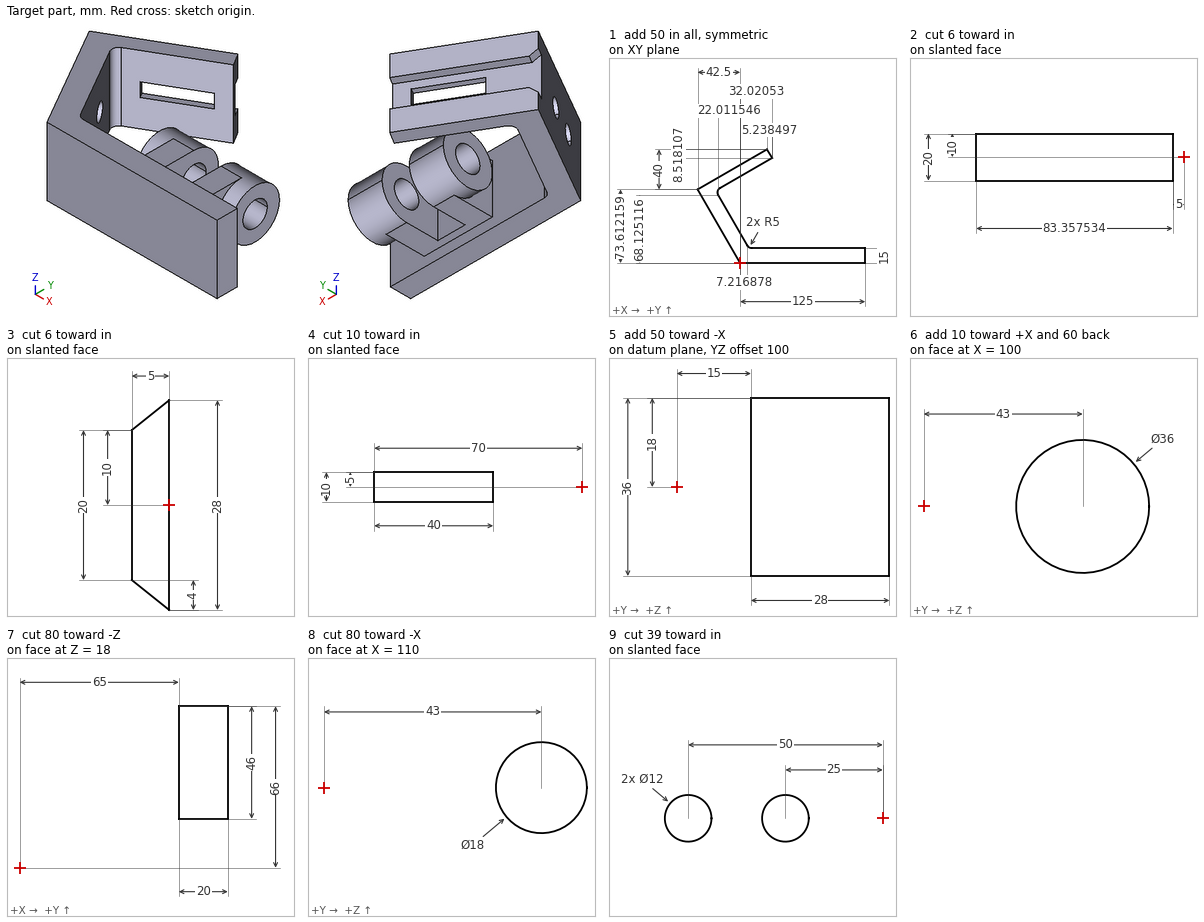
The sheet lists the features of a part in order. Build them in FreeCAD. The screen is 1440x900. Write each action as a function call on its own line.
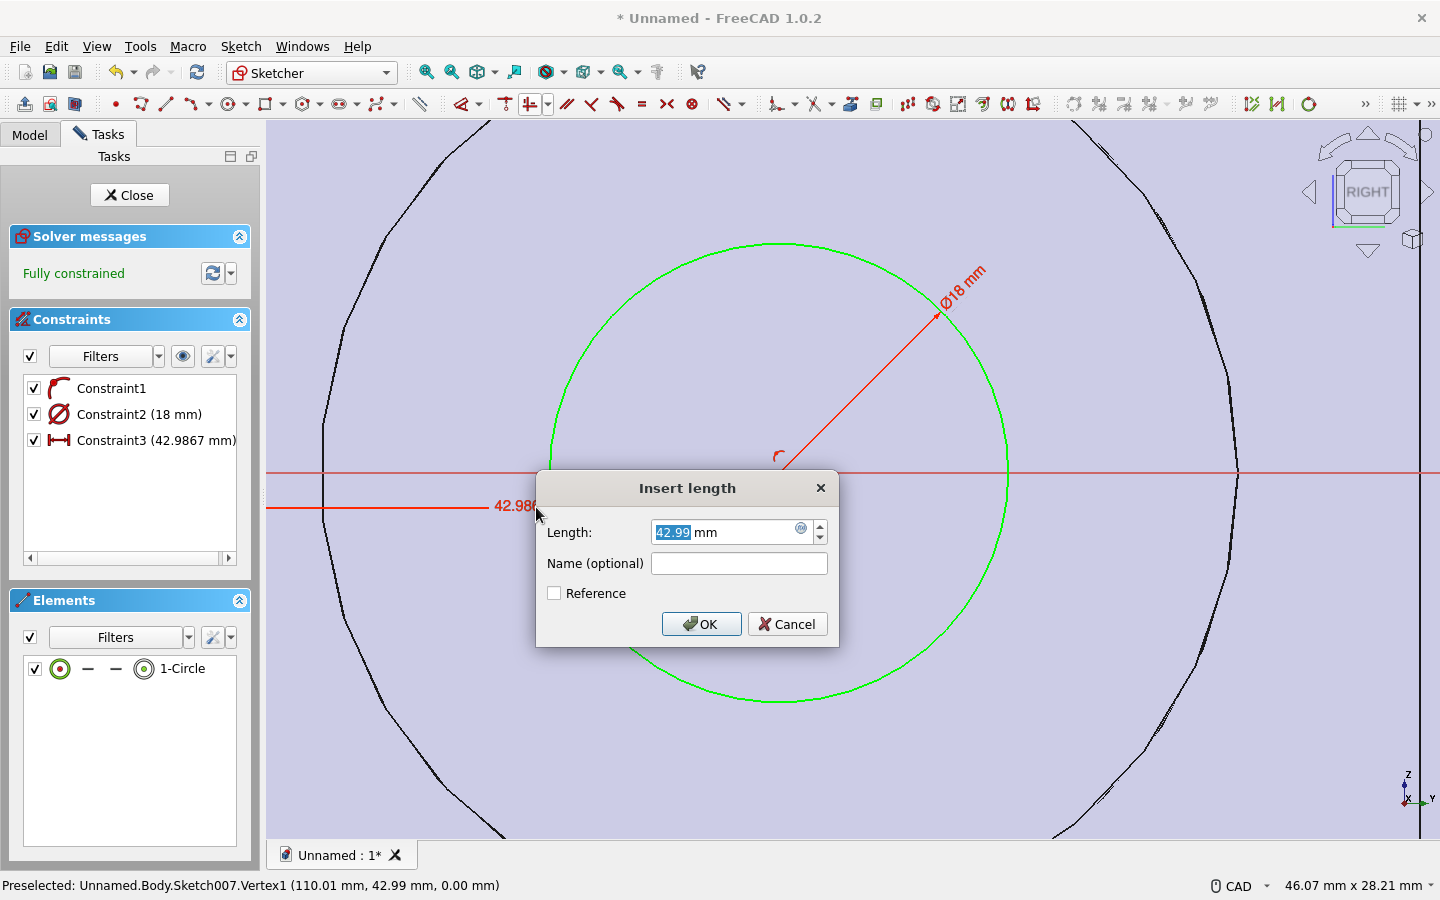
text(43)
key(Return)
key(Escape)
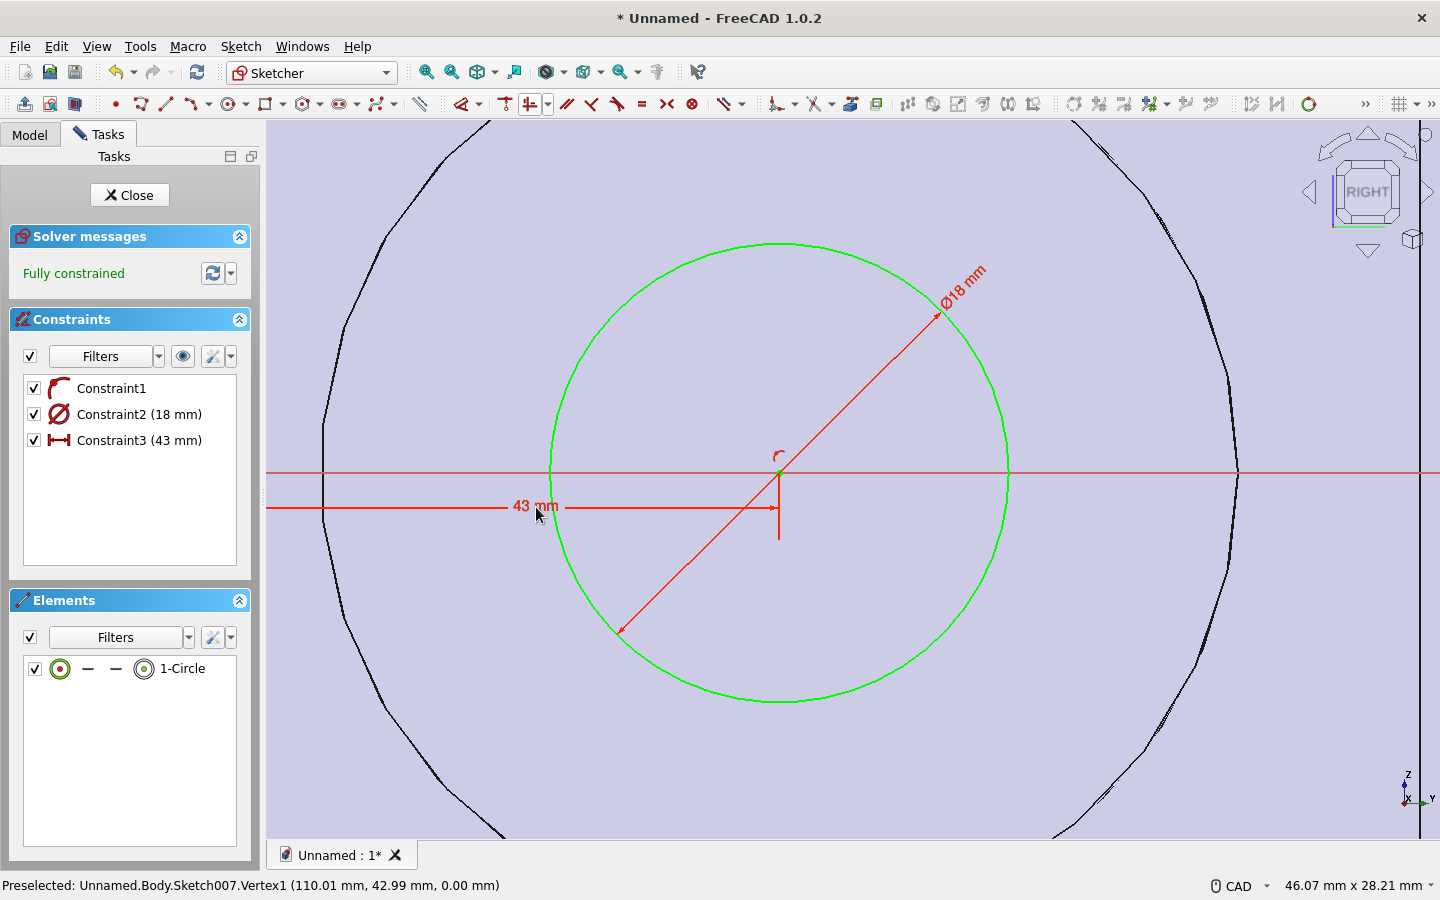
click(130, 195)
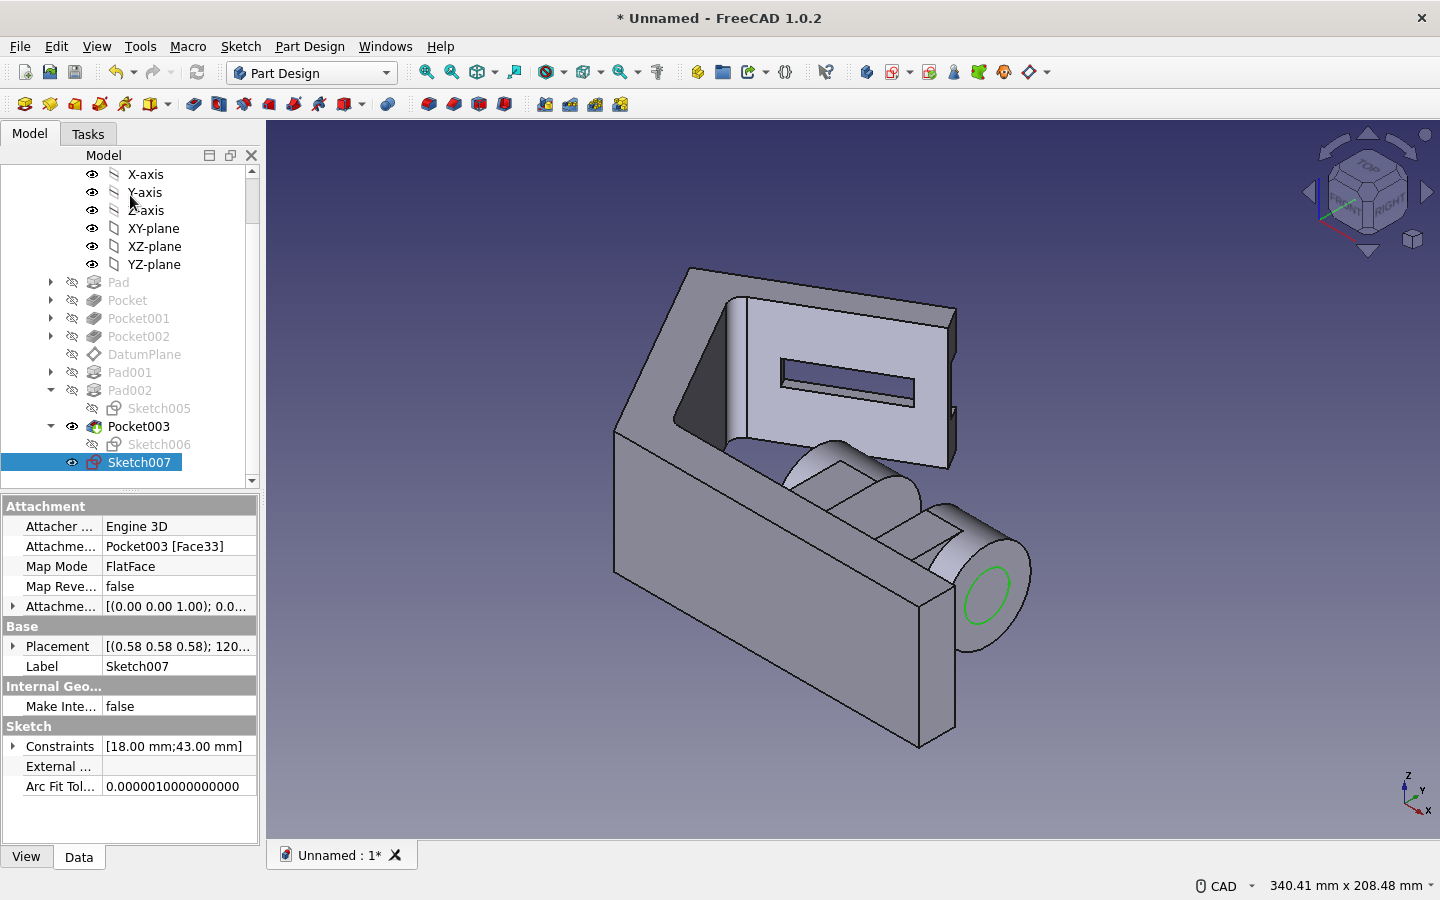
click(194, 104)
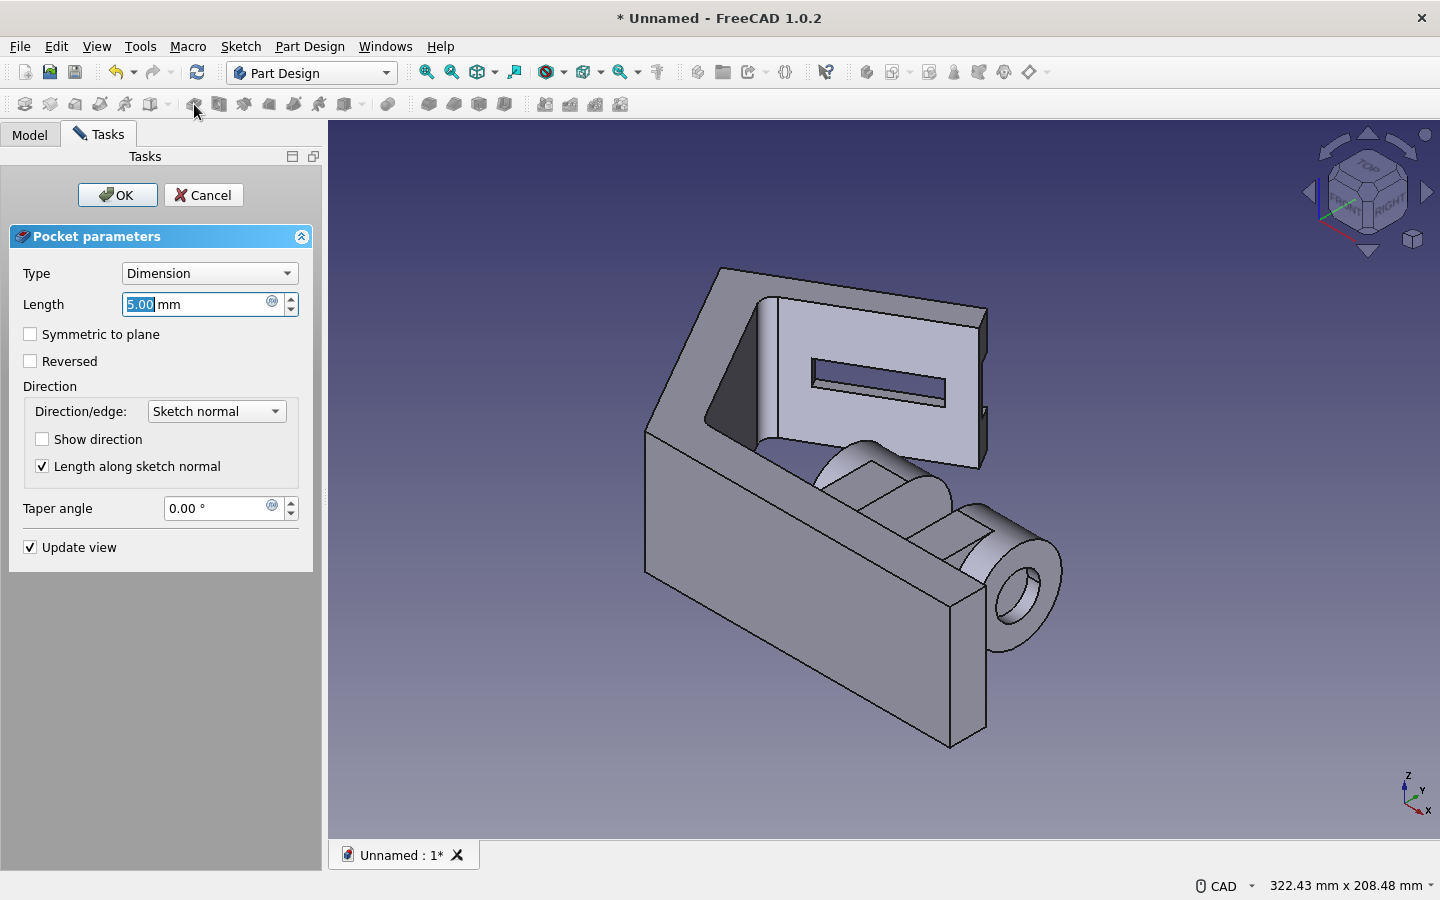
text(80)
key(Tab)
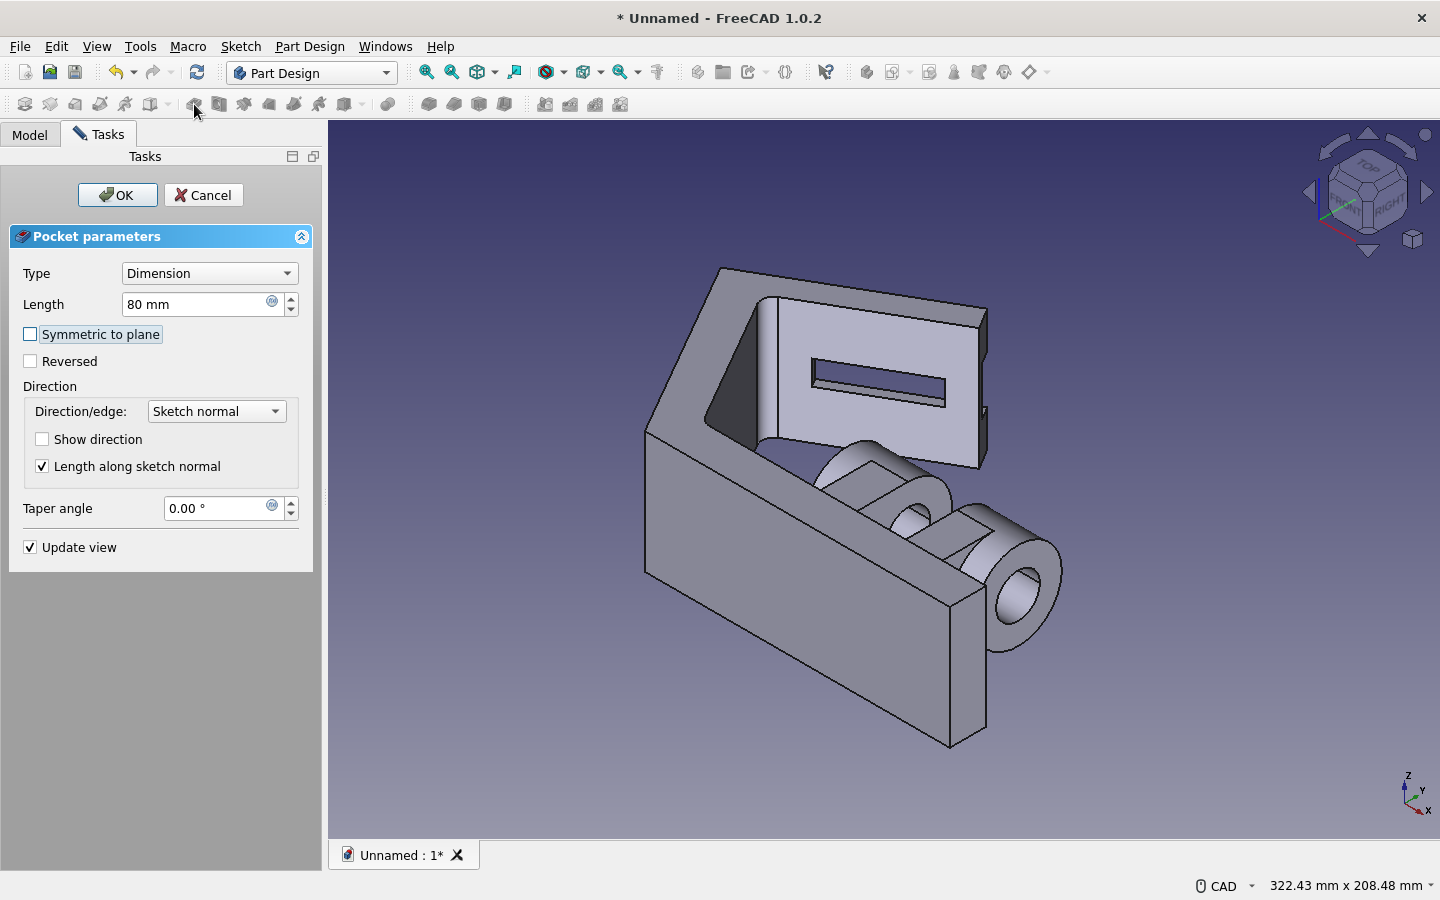
click(118, 195)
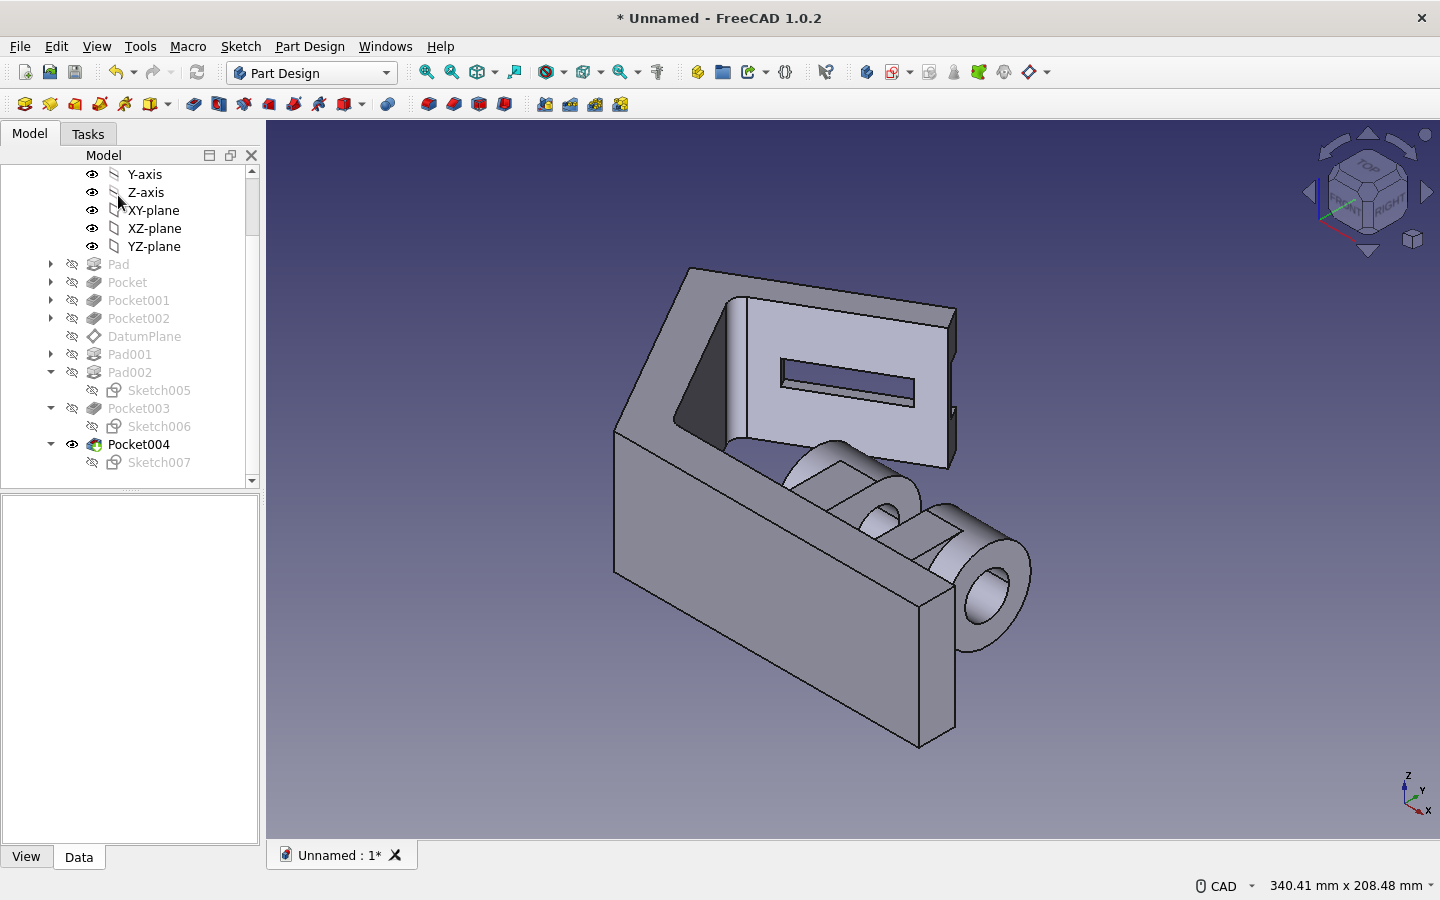
key(6)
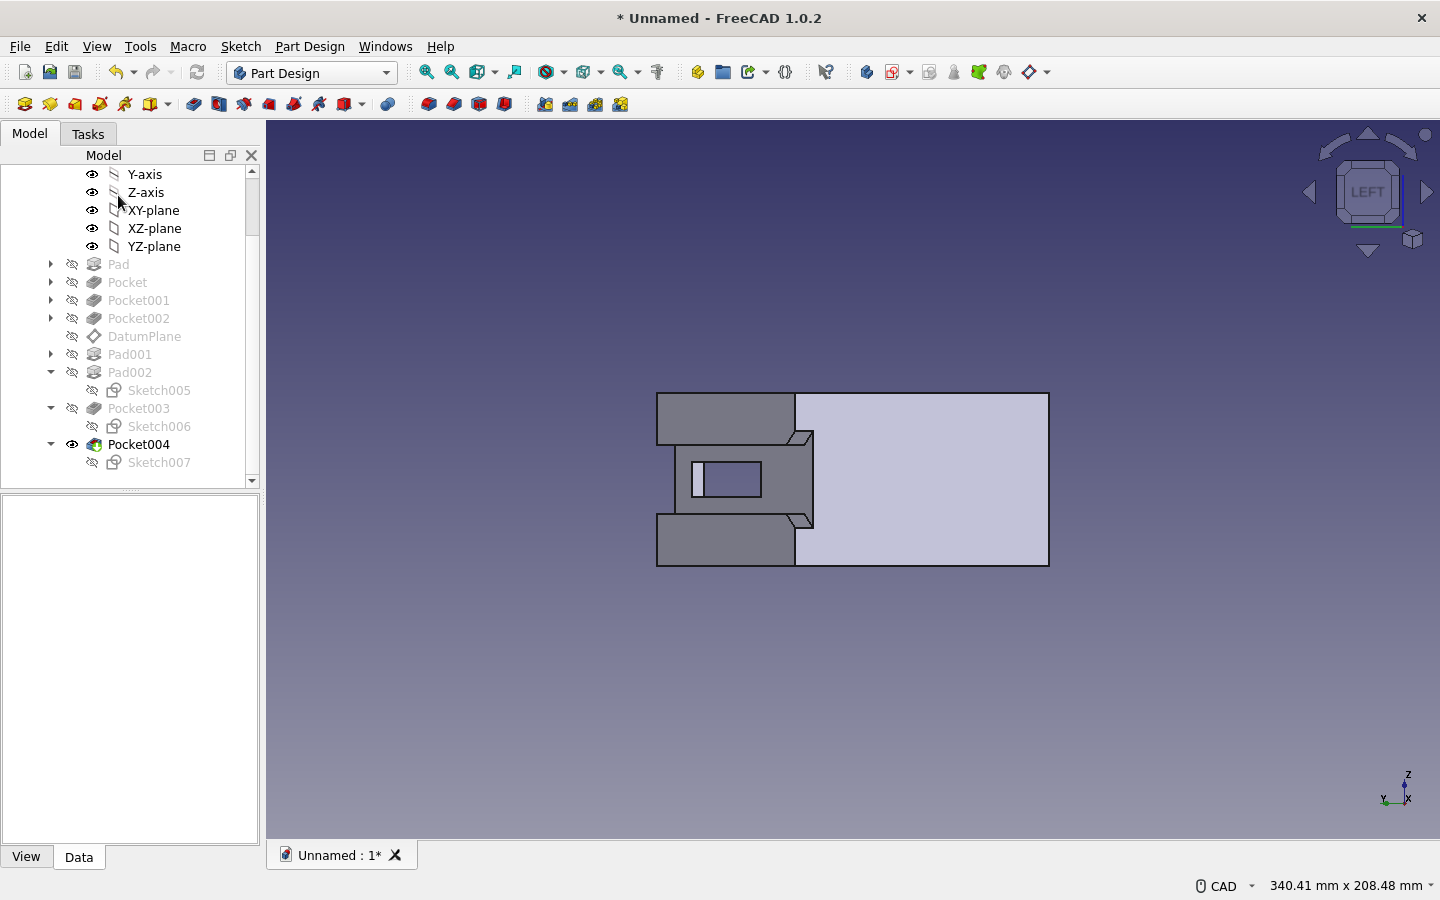
key(v)
key(f)